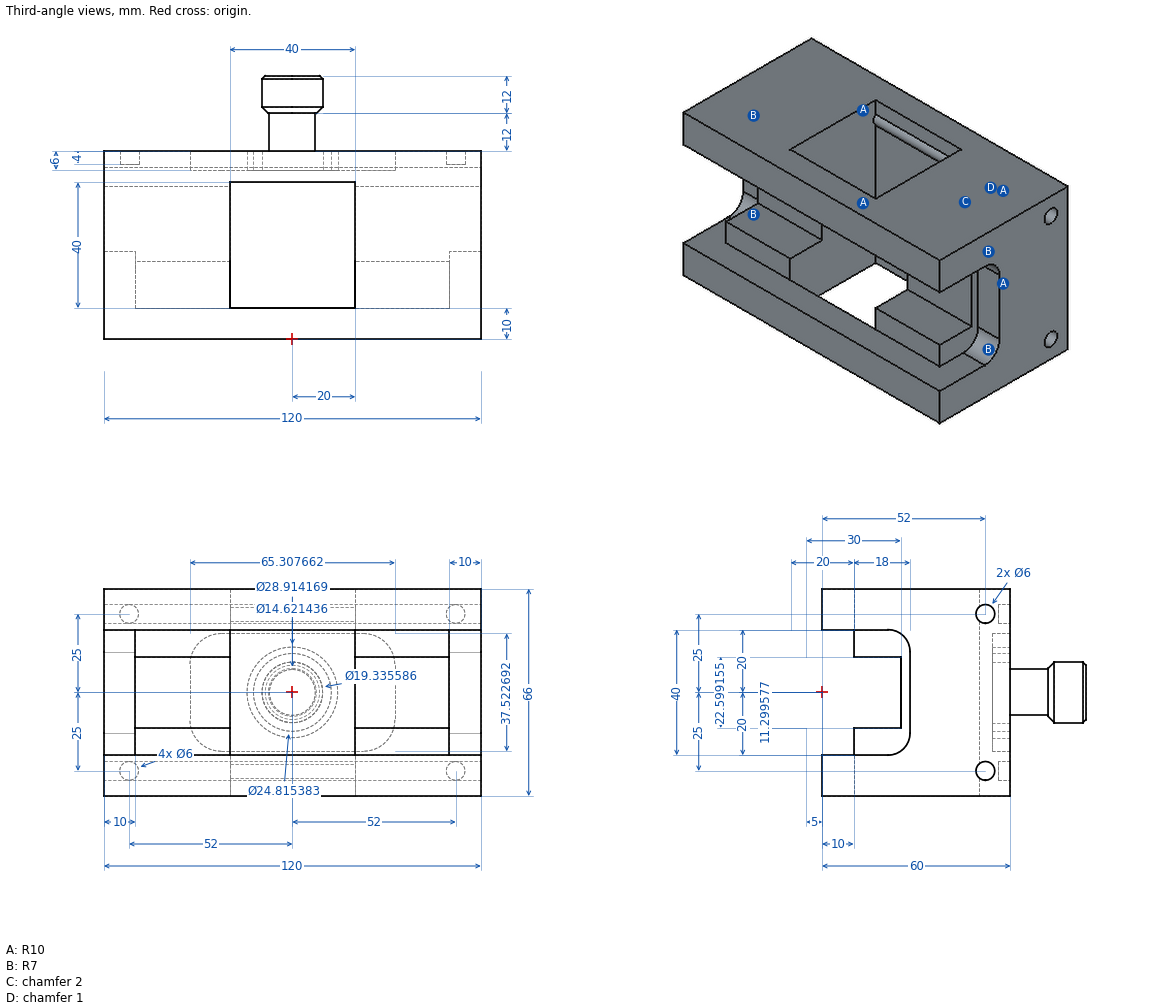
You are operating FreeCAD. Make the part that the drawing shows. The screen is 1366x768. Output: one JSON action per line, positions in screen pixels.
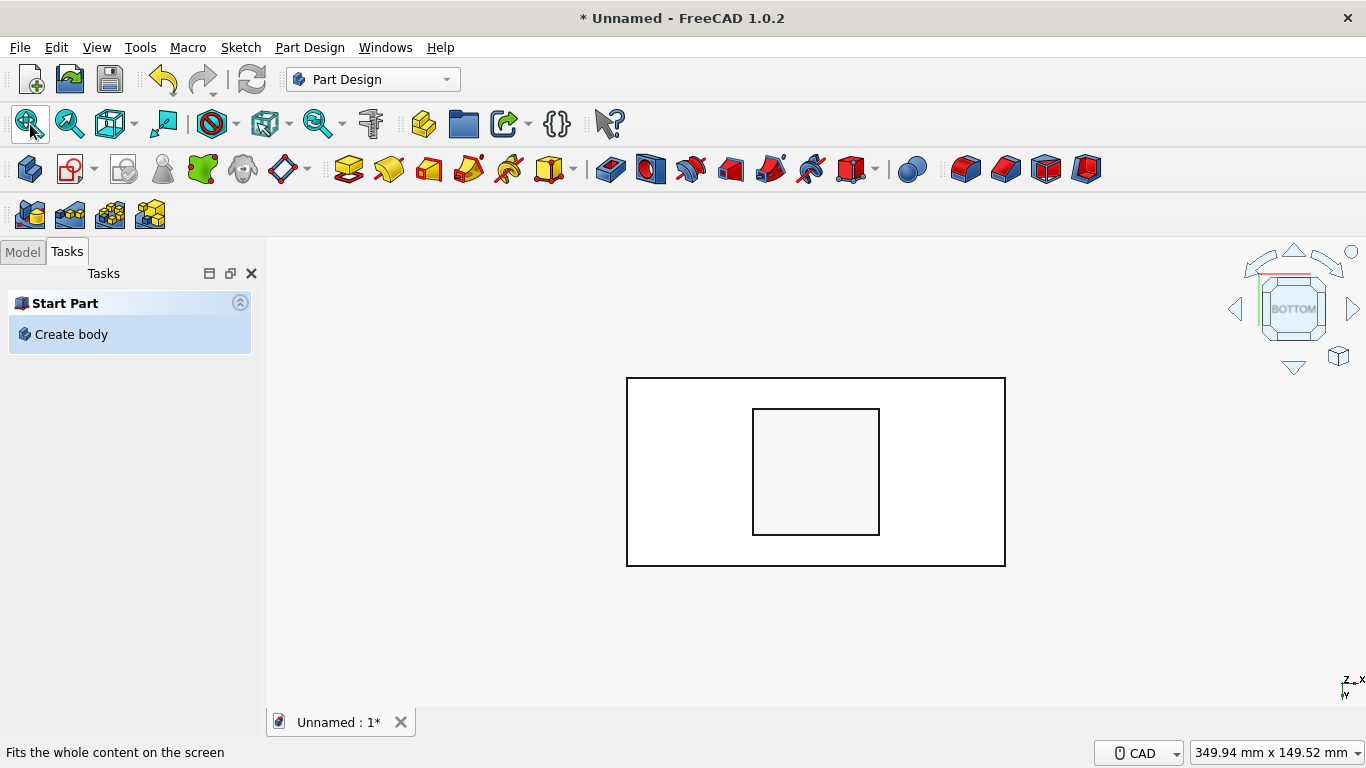
{"action": "key", "text": "4"}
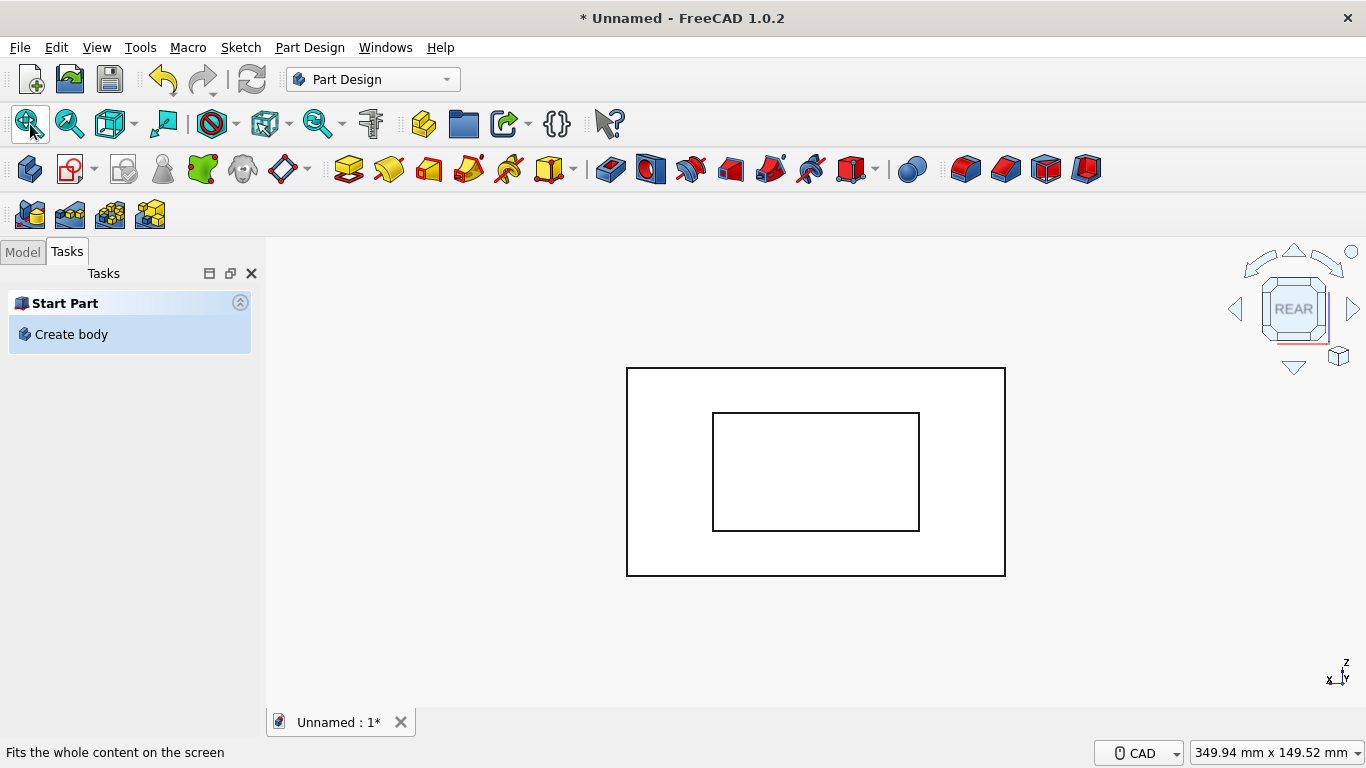
{"action": "left_click", "coordinate": [30, 124]}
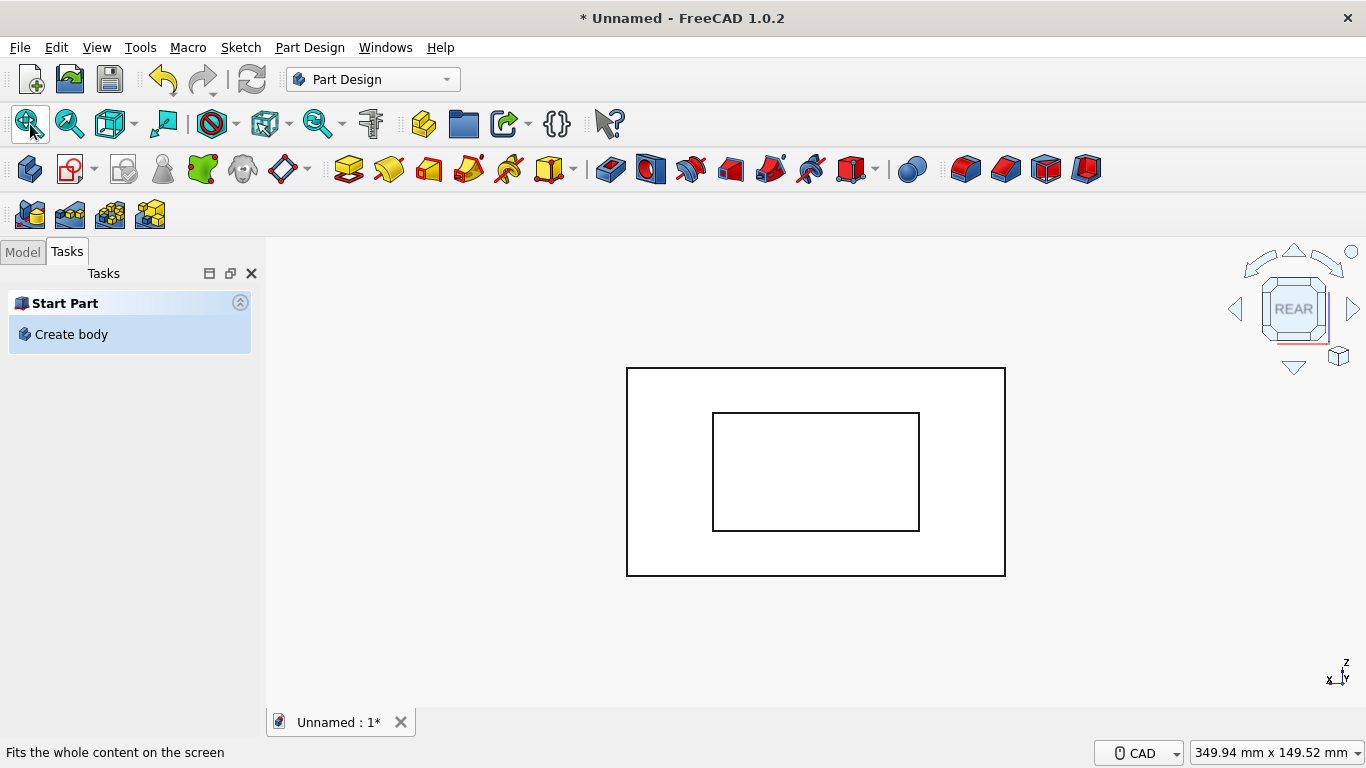
{"action": "scroll", "coordinate": [713, 530], "scroll_direction": "up", "scroll_amount": 4}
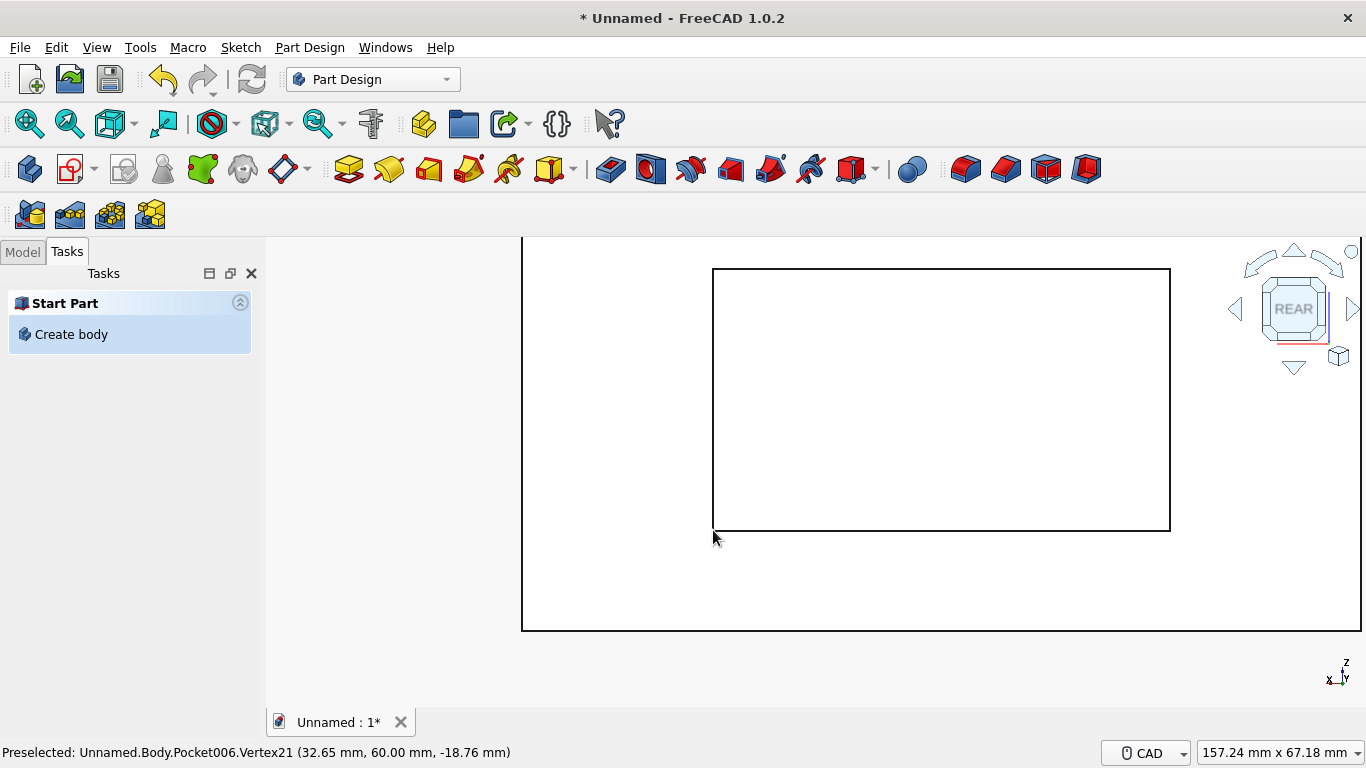
{"action": "left_click", "coordinate": [30, 124]}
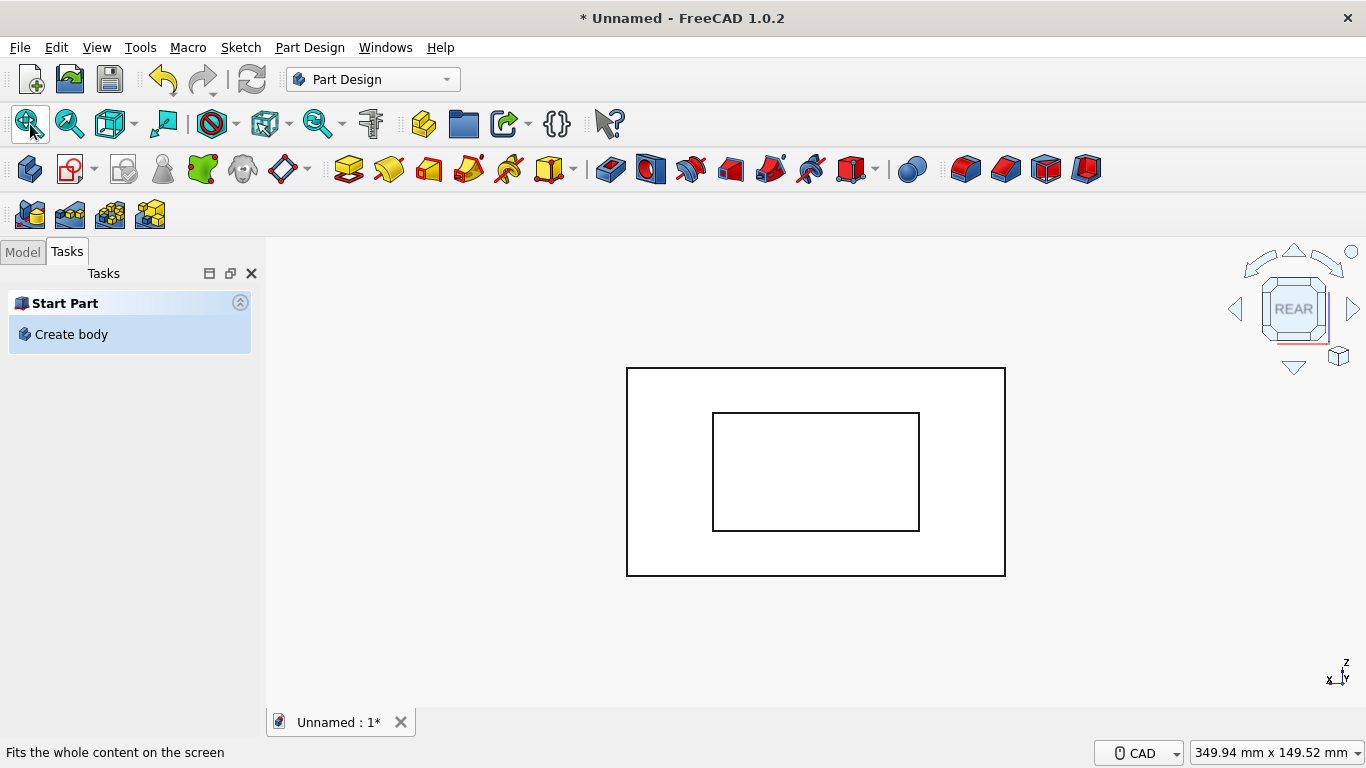
{"action": "key", "text": "6"}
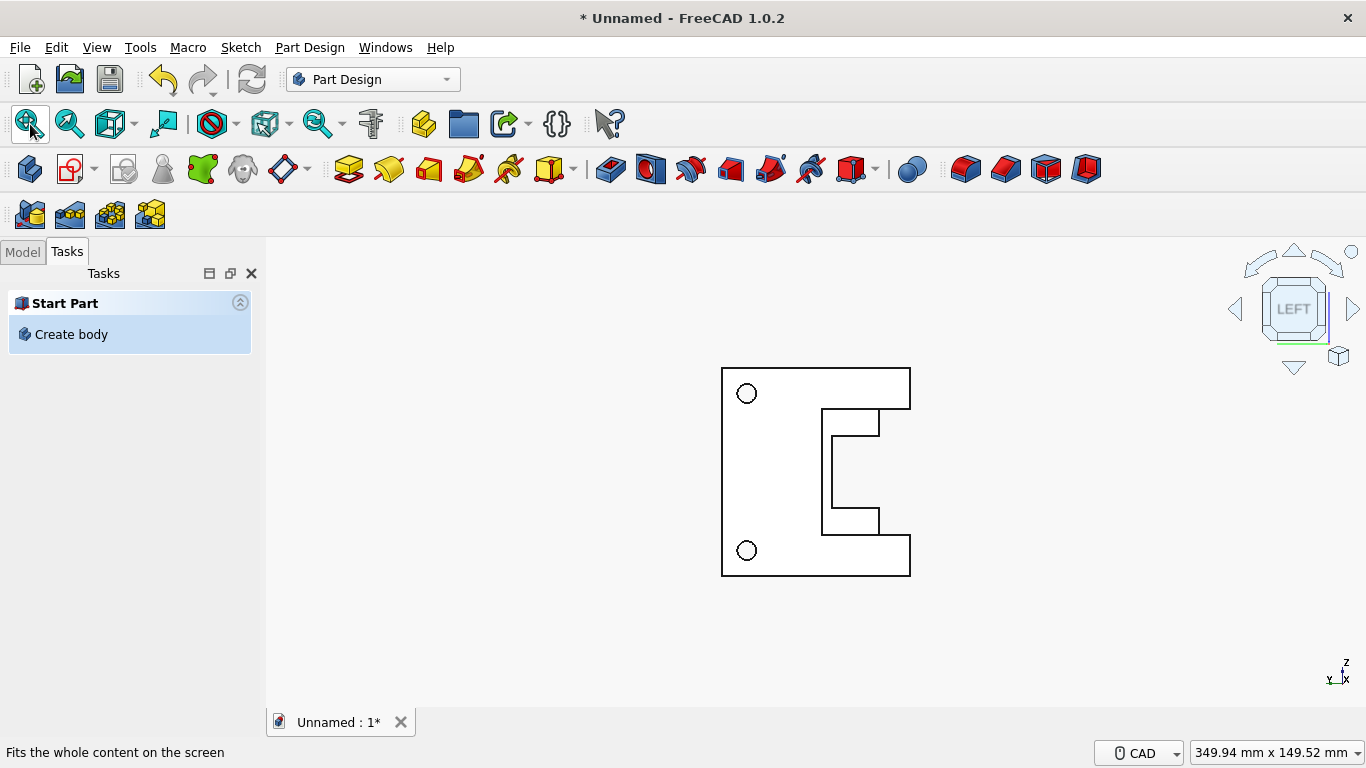
{"action": "left_click", "coordinate": [30, 124]}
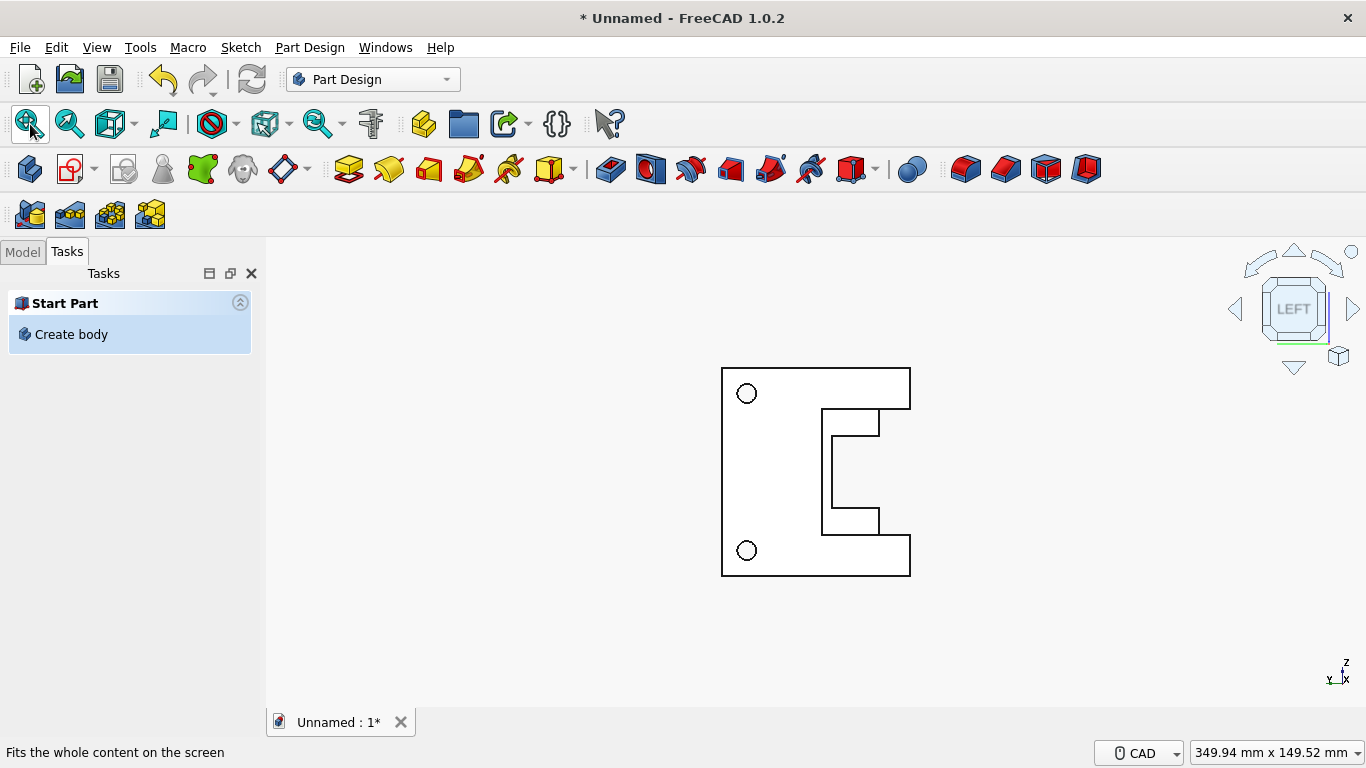
{"action": "scroll", "coordinate": [731, 530], "scroll_direction": "up", "scroll_amount": 4}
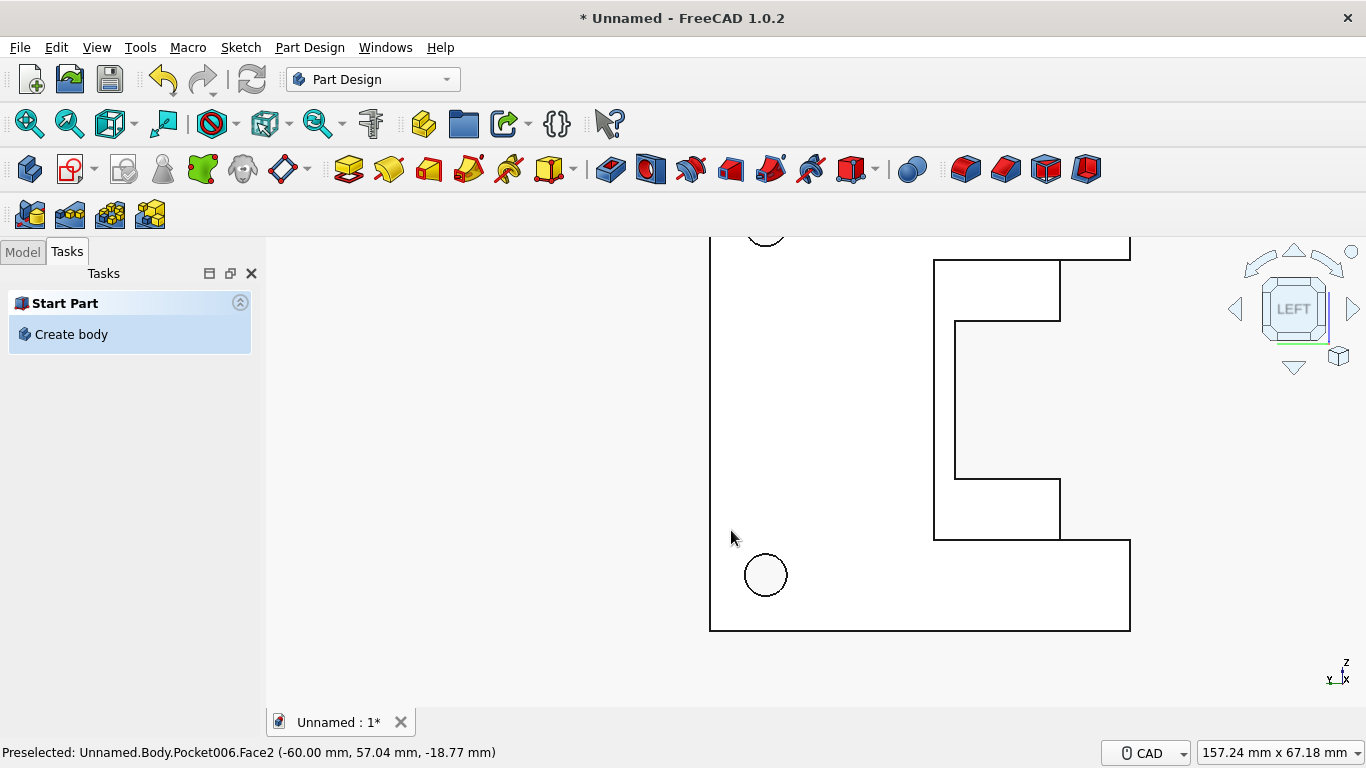
{"action": "left_click", "coordinate": [30, 124]}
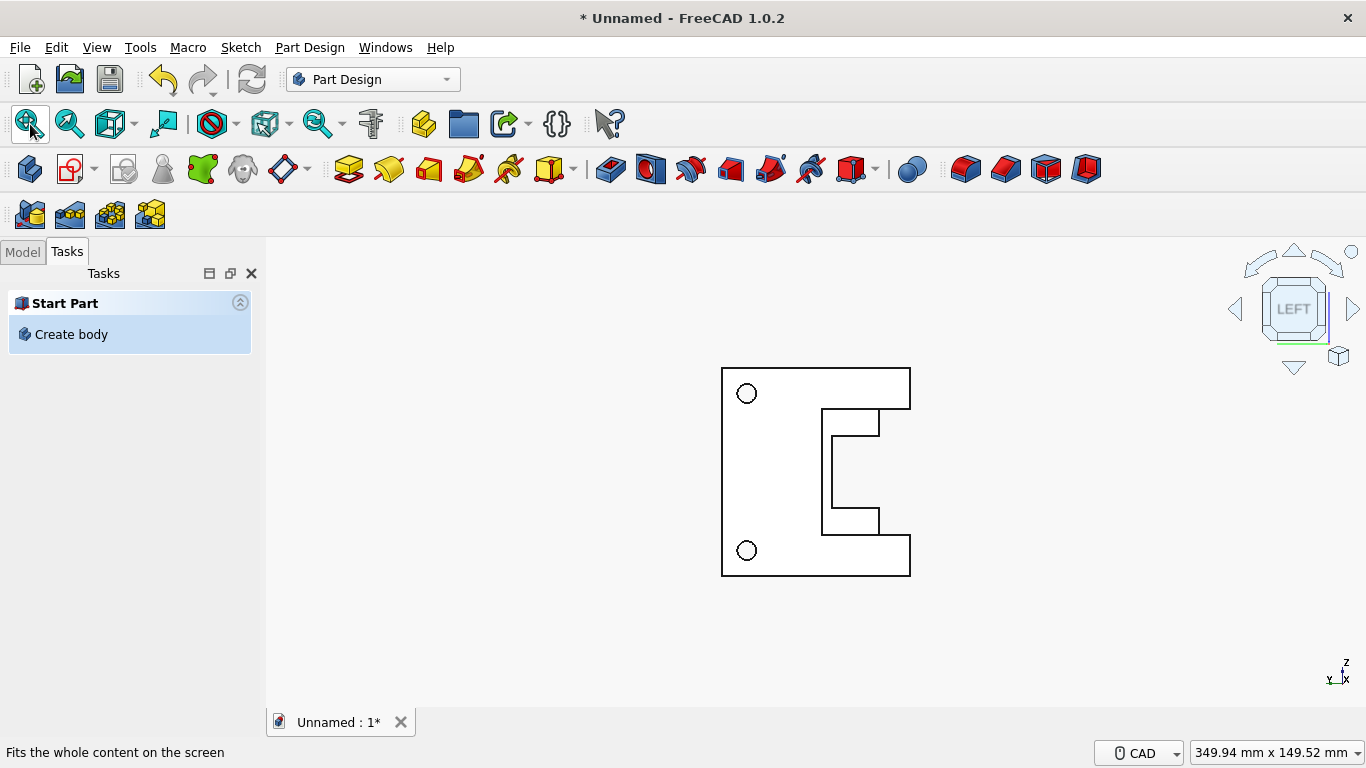
{"action": "key", "text": "v 3"}